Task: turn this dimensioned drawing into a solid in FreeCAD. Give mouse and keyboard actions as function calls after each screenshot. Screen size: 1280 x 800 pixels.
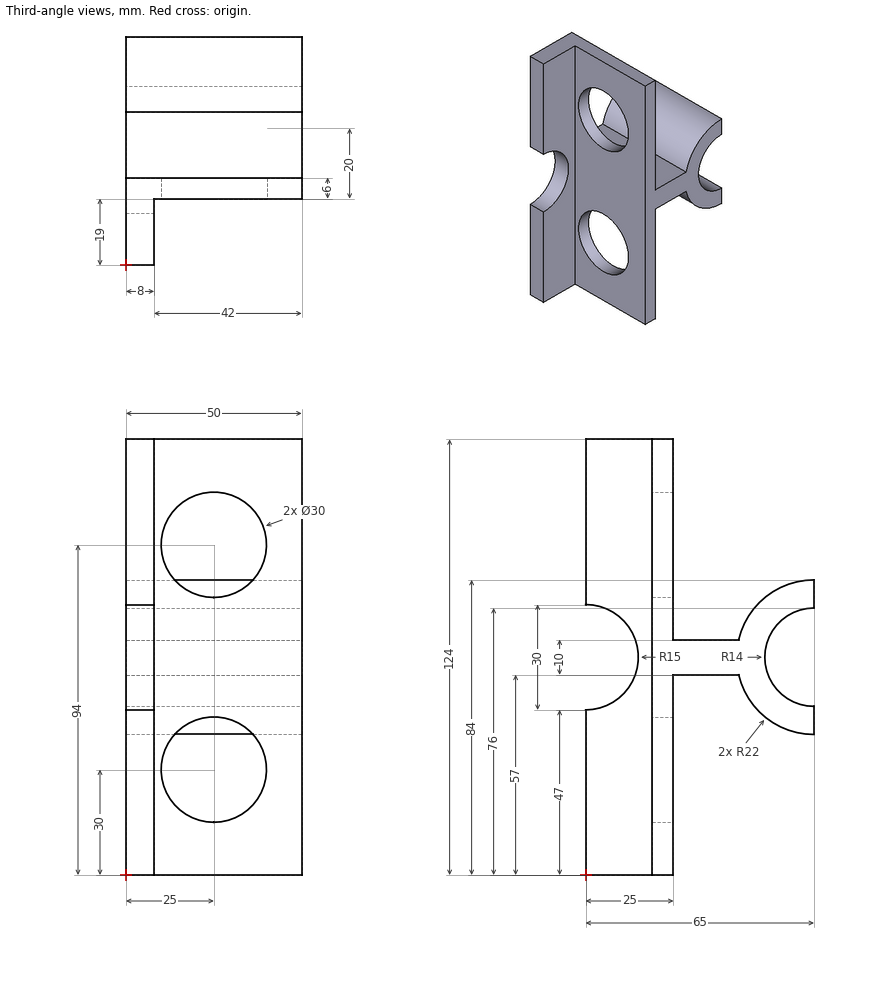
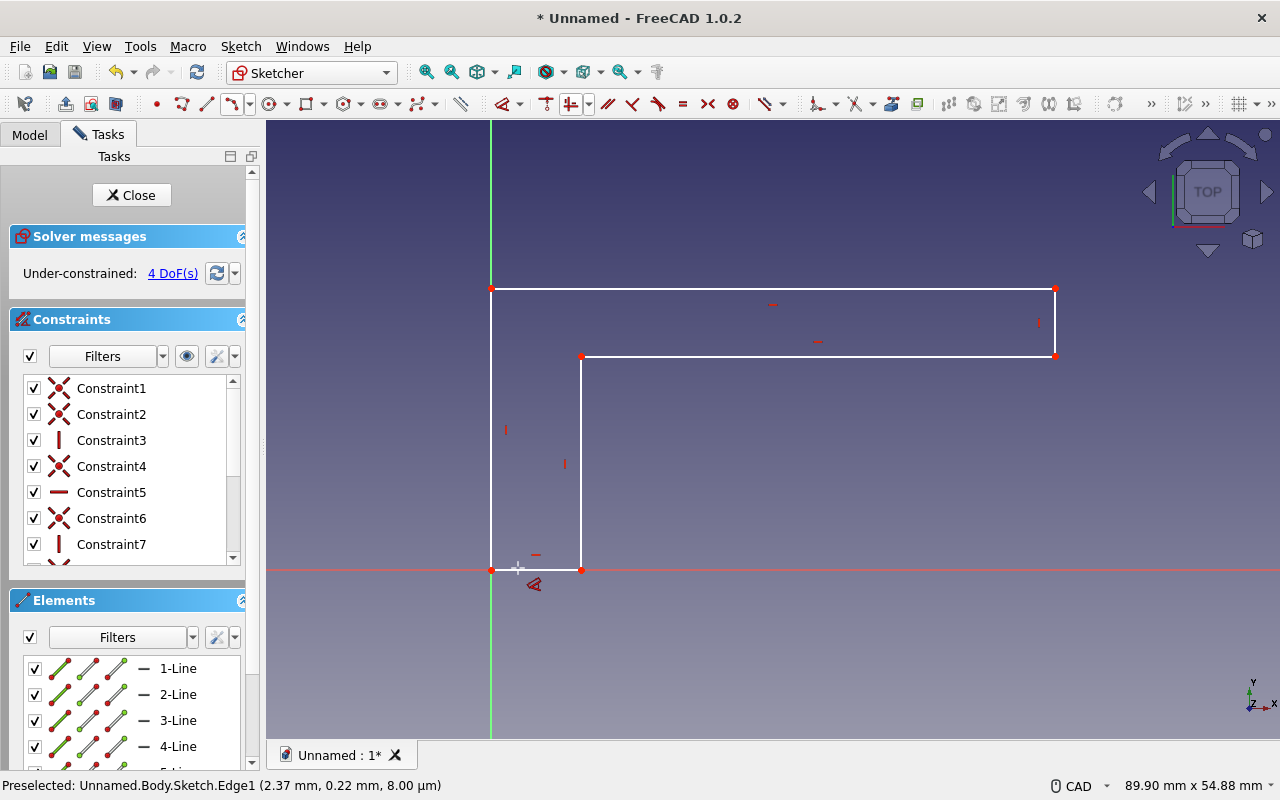
click(518, 570)
click(536, 604)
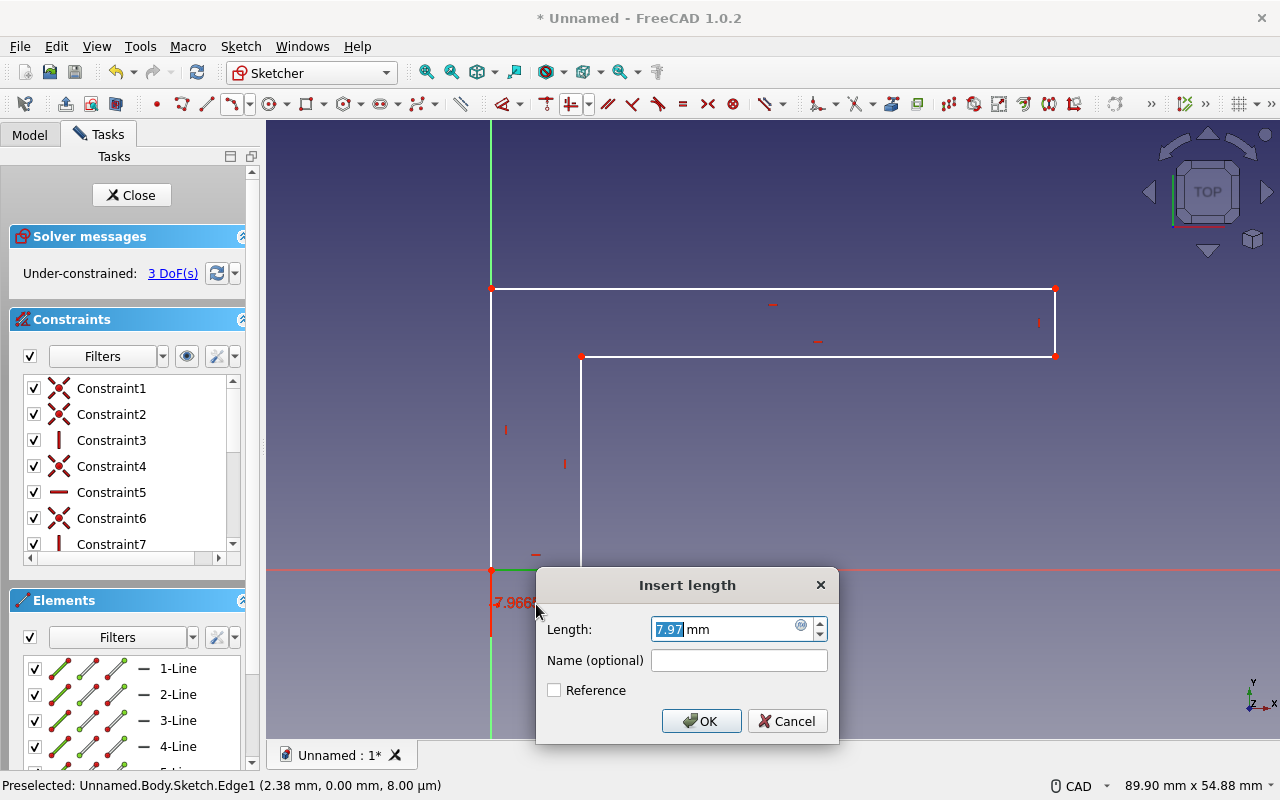
text(8)
key(Return)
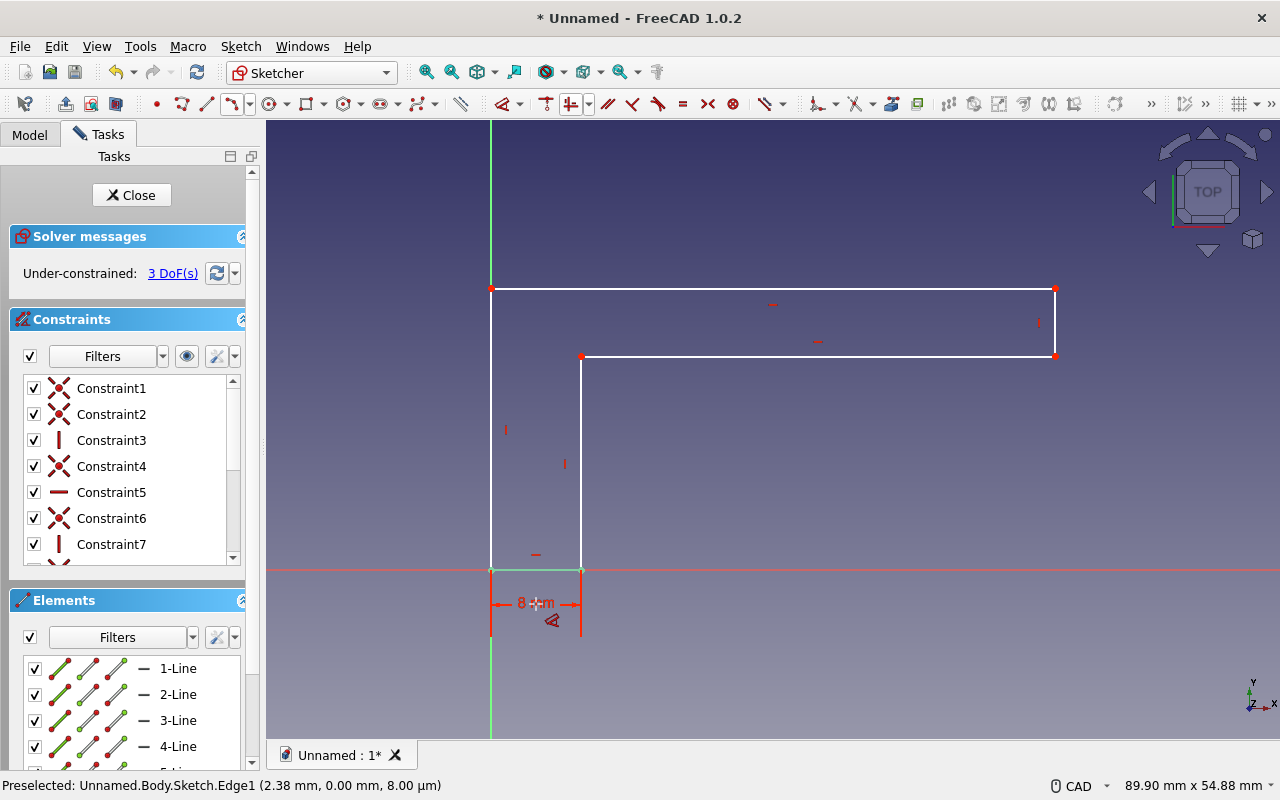
click(1055, 337)
click(1089, 323)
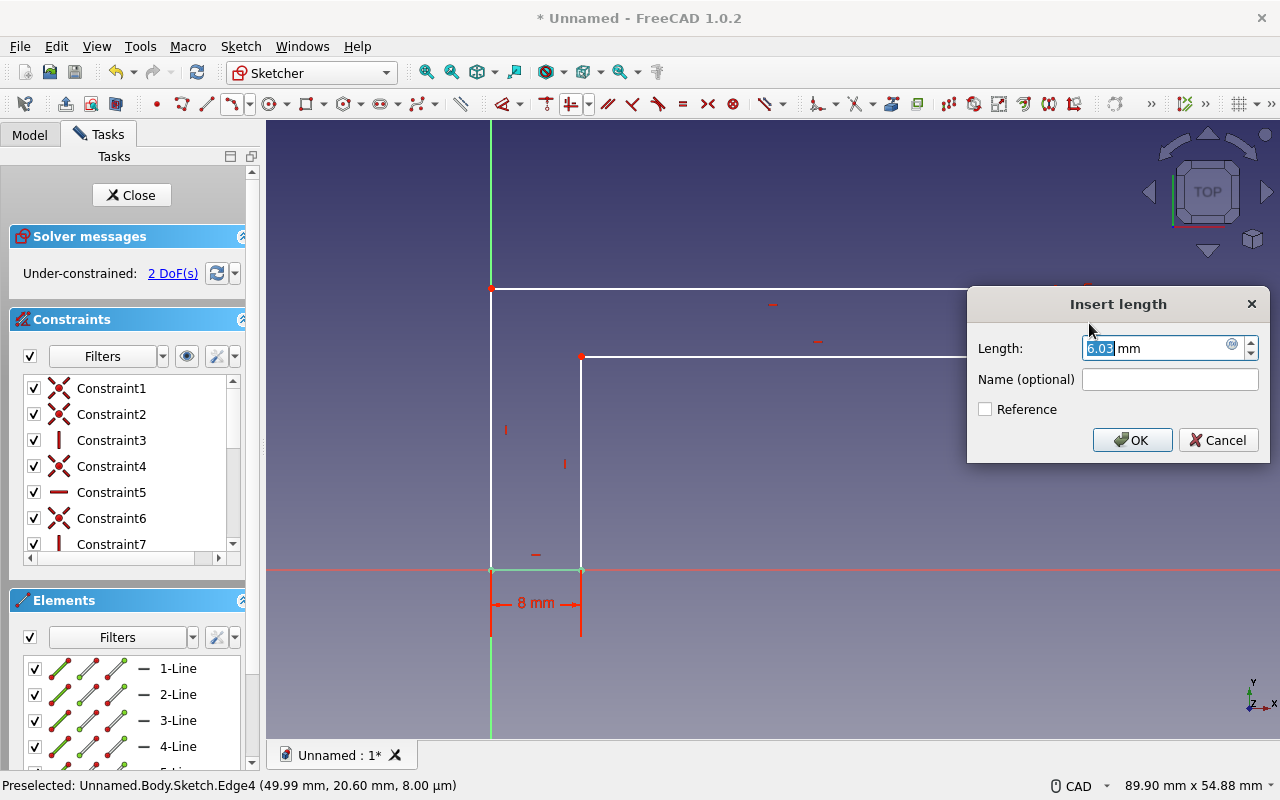
text(6)
key(Return)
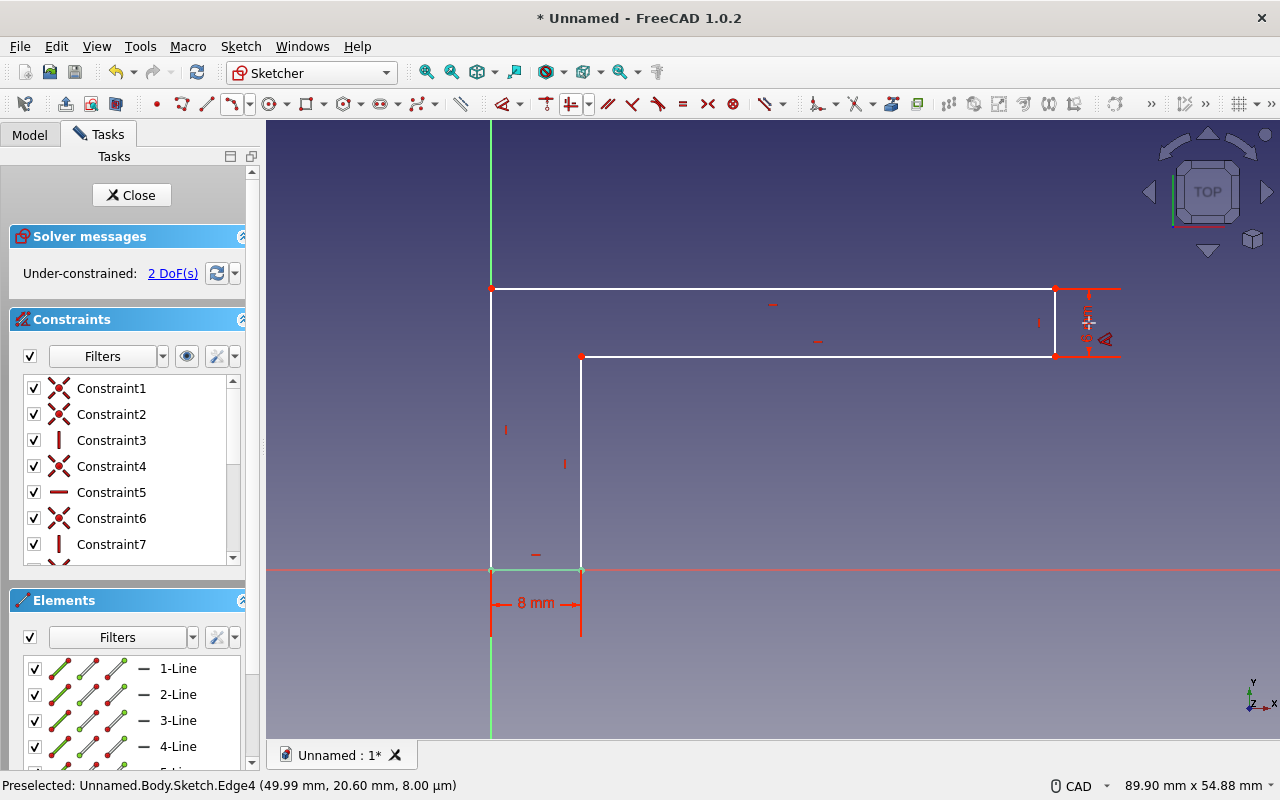
click(581, 506)
click(547, 463)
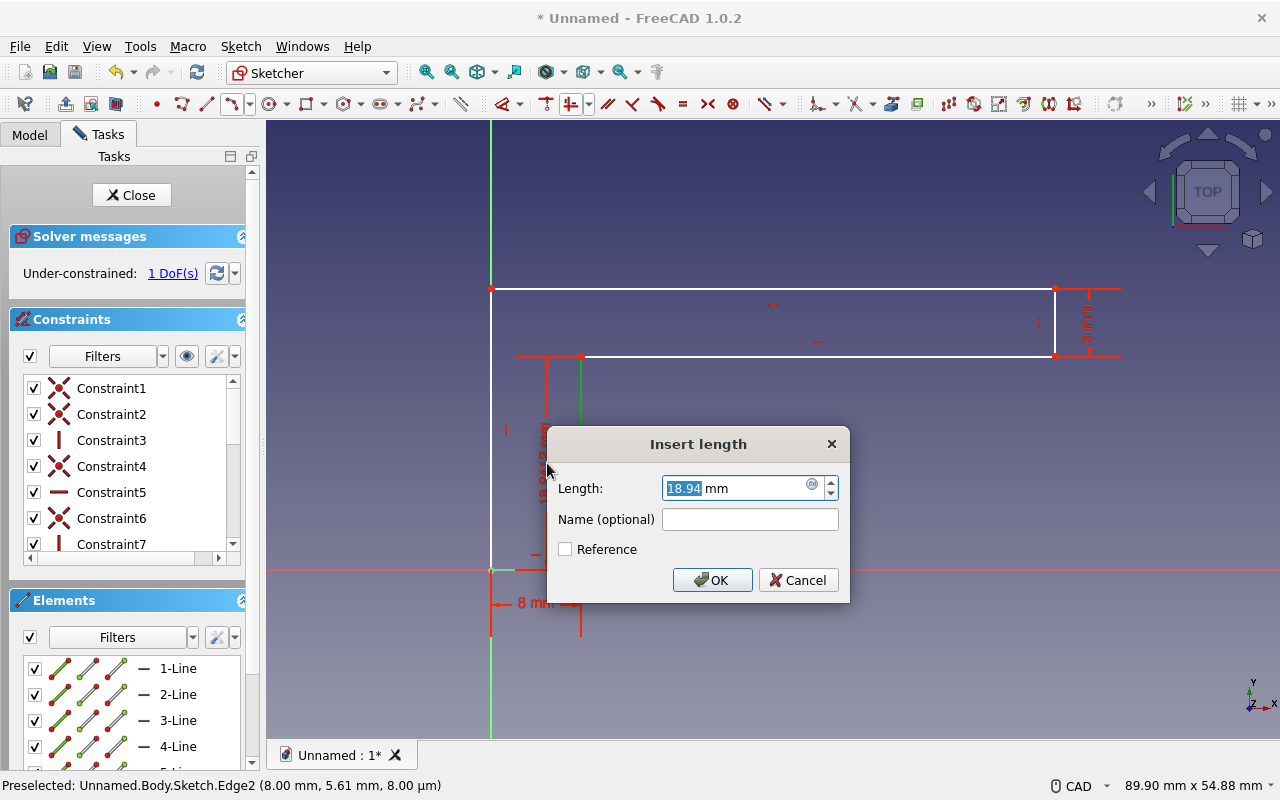
text(19)
key(Return)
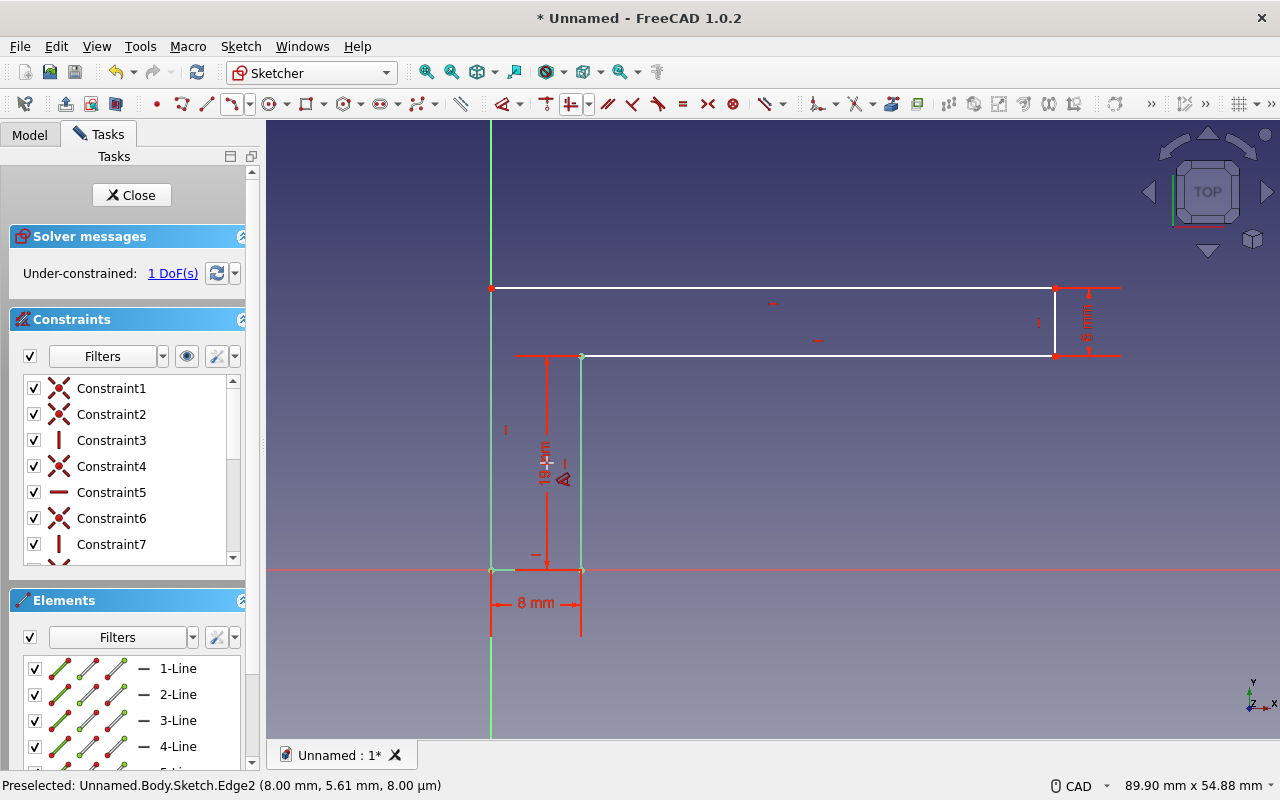
click(723, 356)
click(818, 322)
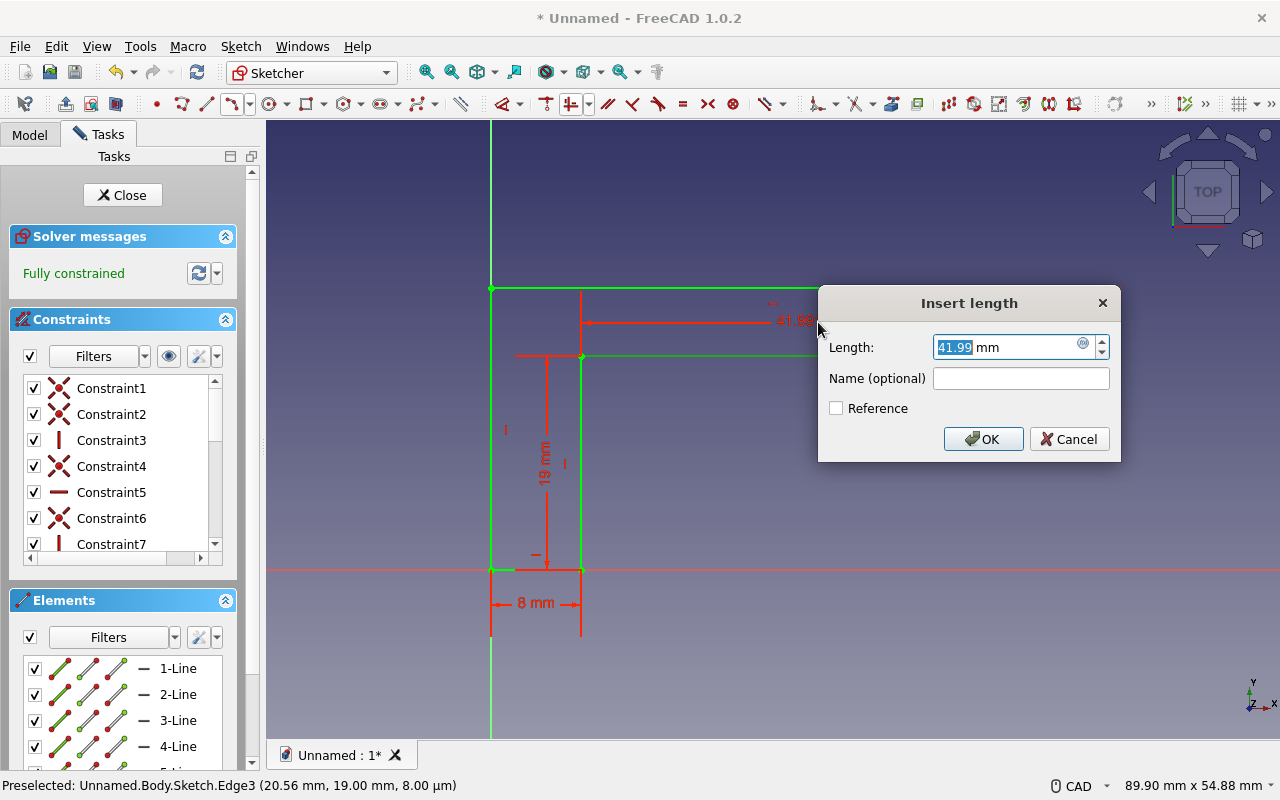
text(42)
key(Return)
key(Escape)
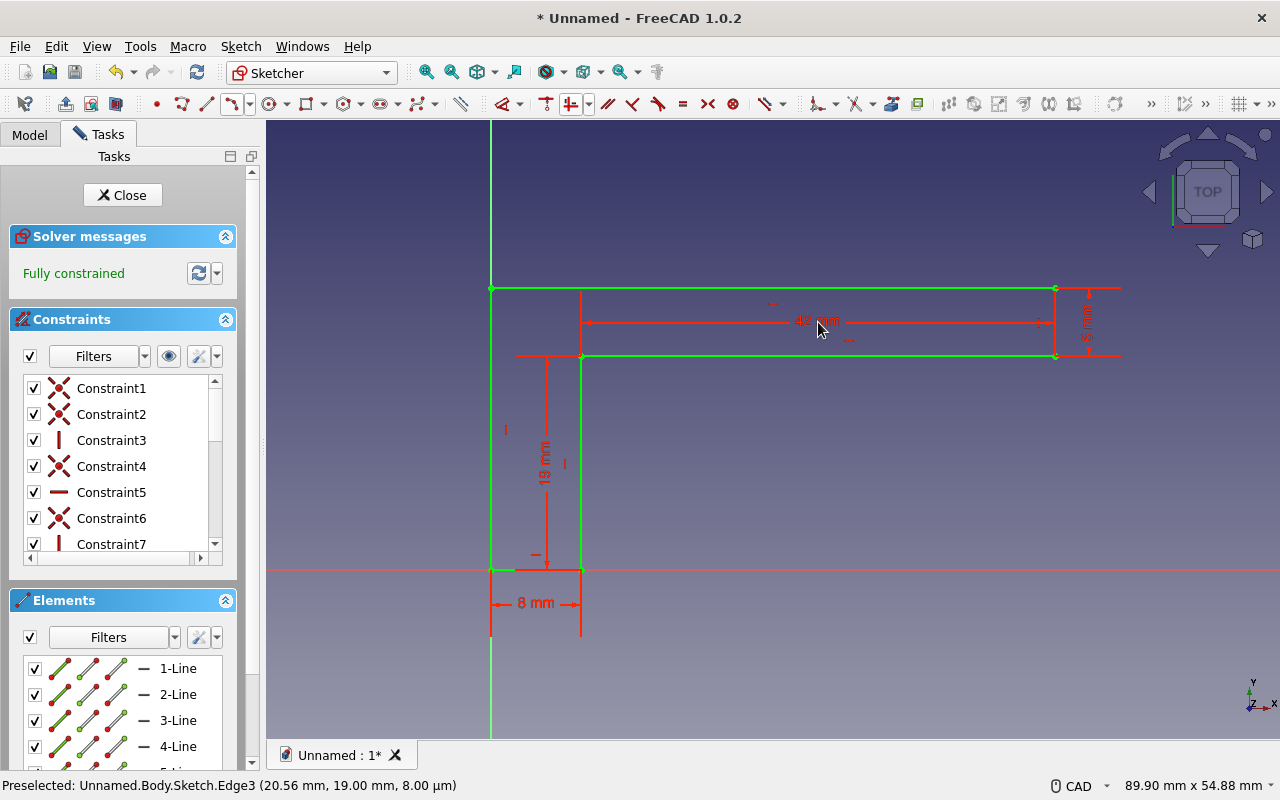
click(123, 195)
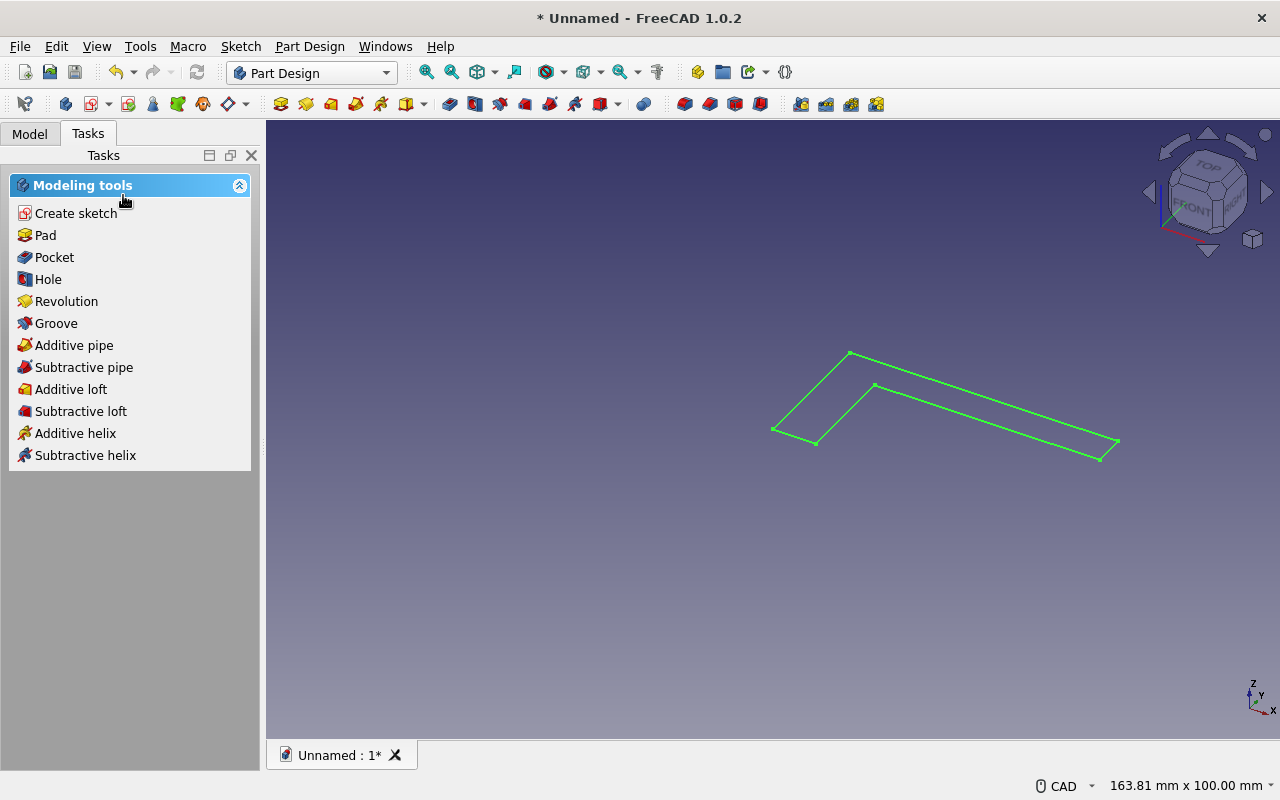
click(281, 104)